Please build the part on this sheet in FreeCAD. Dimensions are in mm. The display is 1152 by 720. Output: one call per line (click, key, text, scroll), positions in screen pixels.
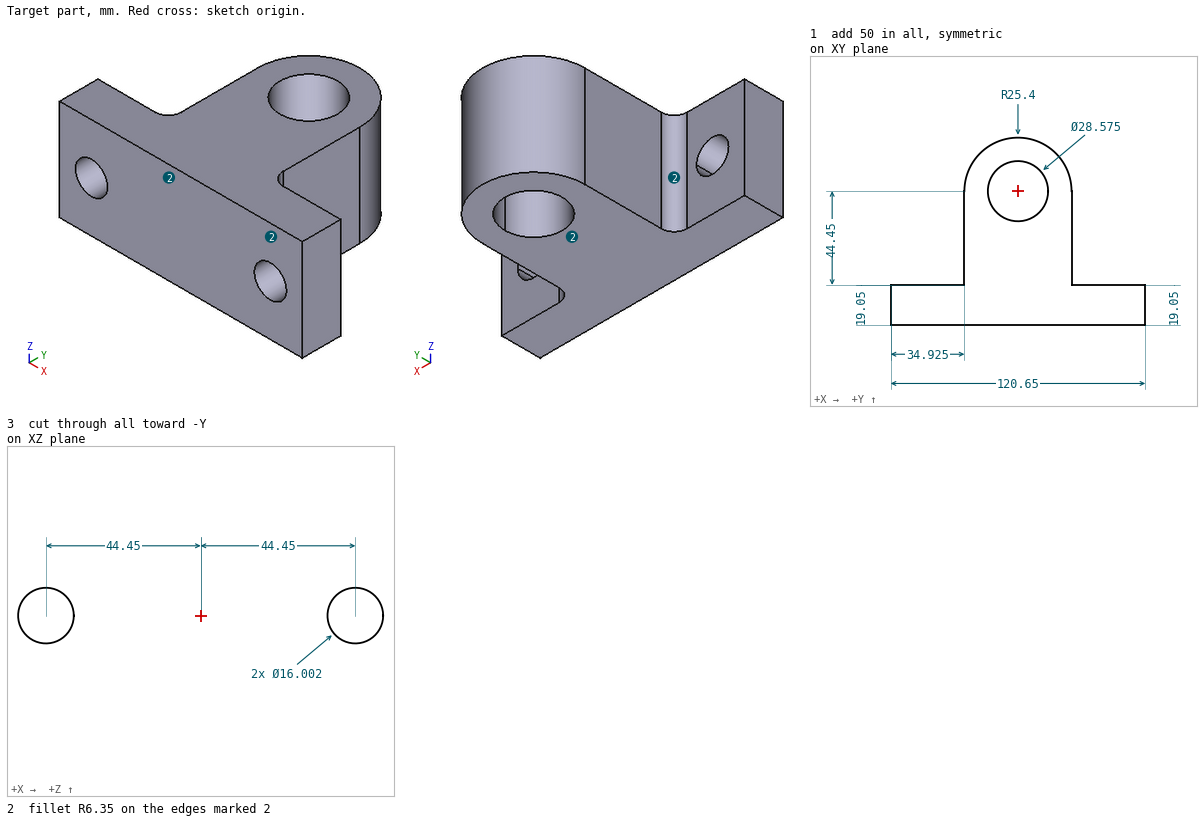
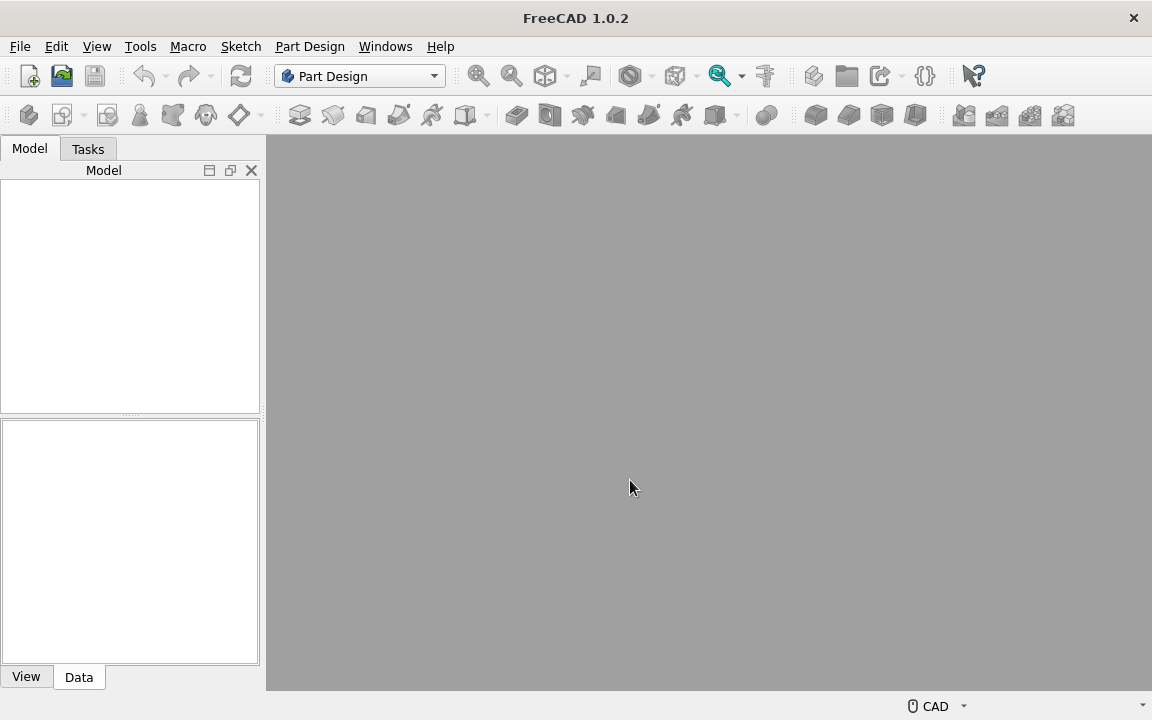
key(ctrl+n)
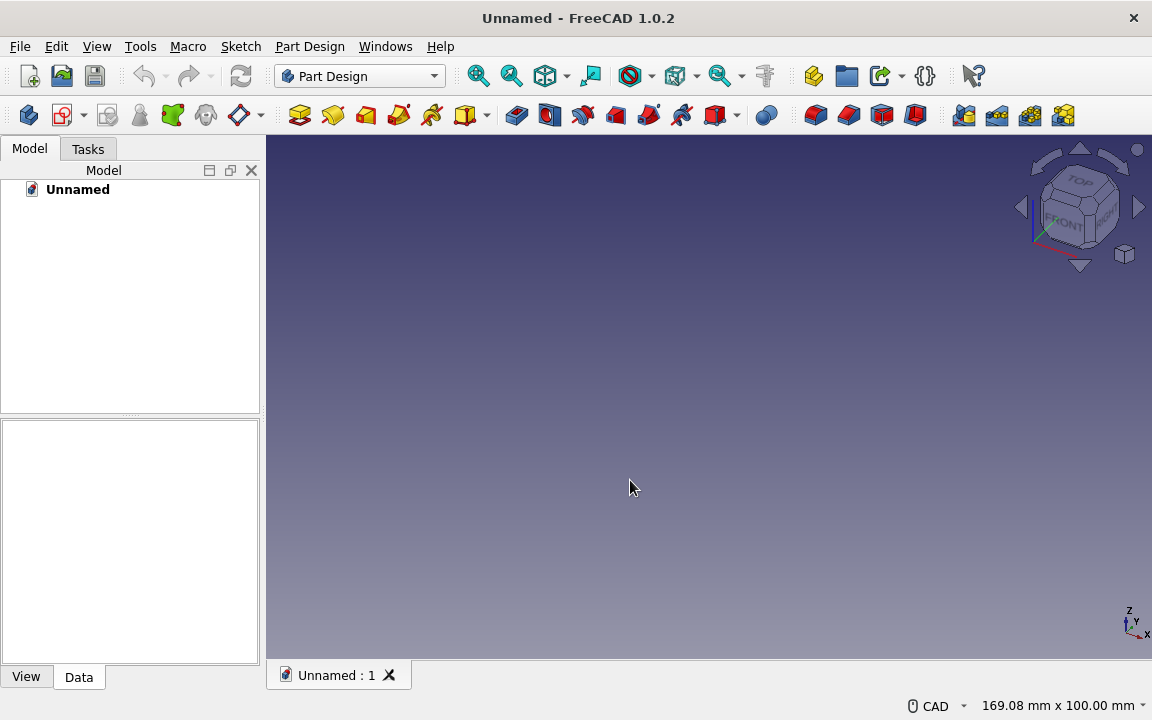
click(62, 116)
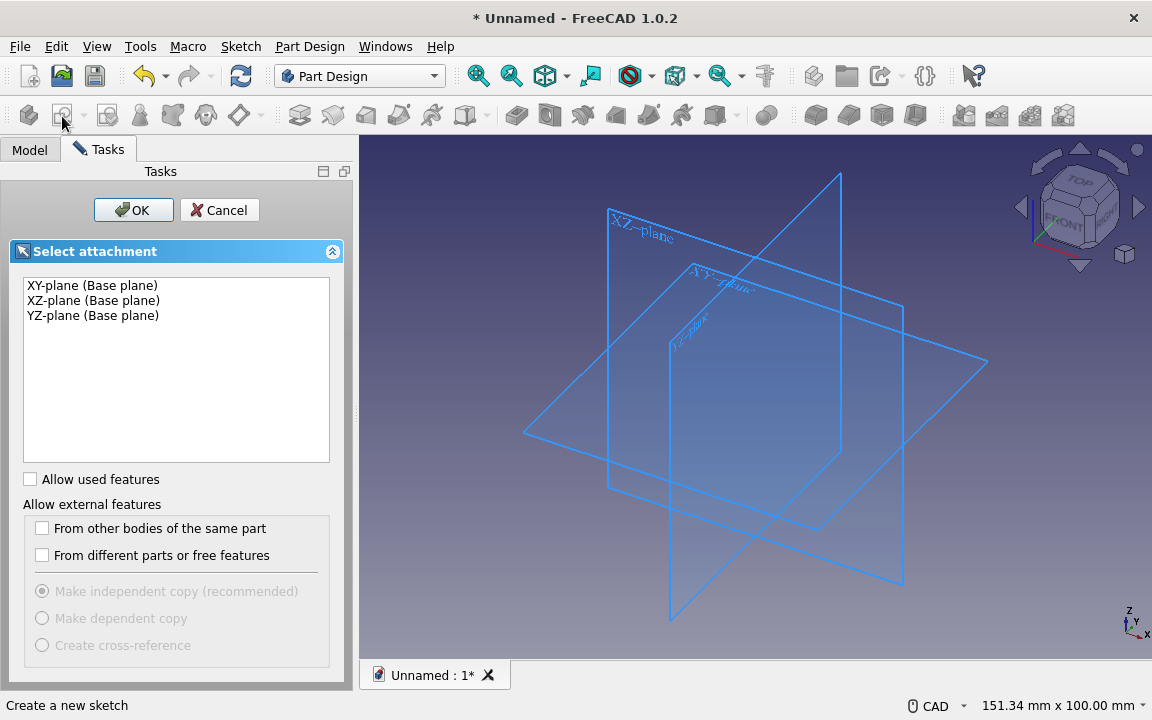
click(84, 286)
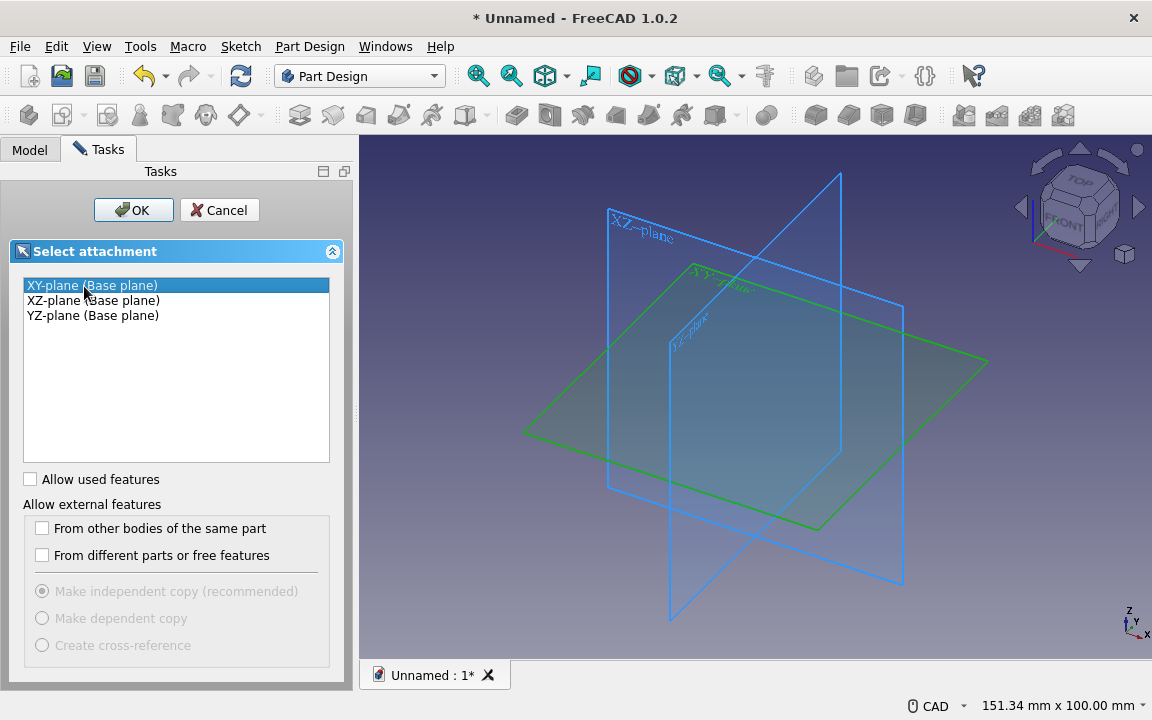
click(134, 210)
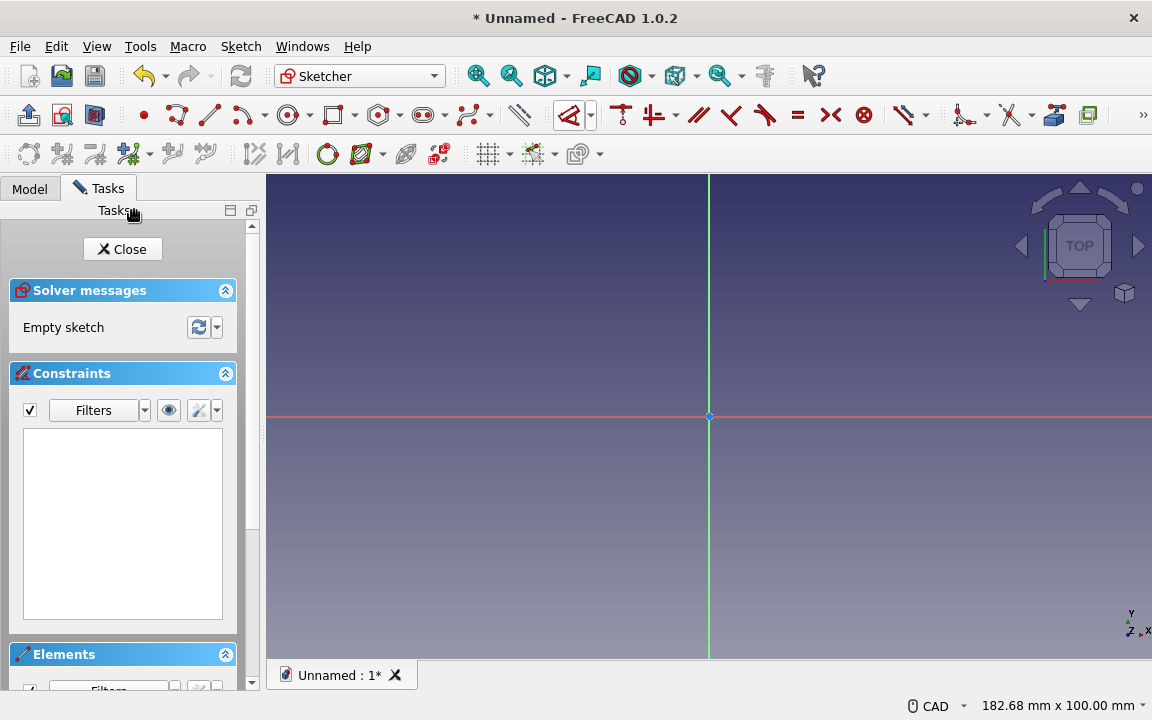
scroll(501, 229, down, 2)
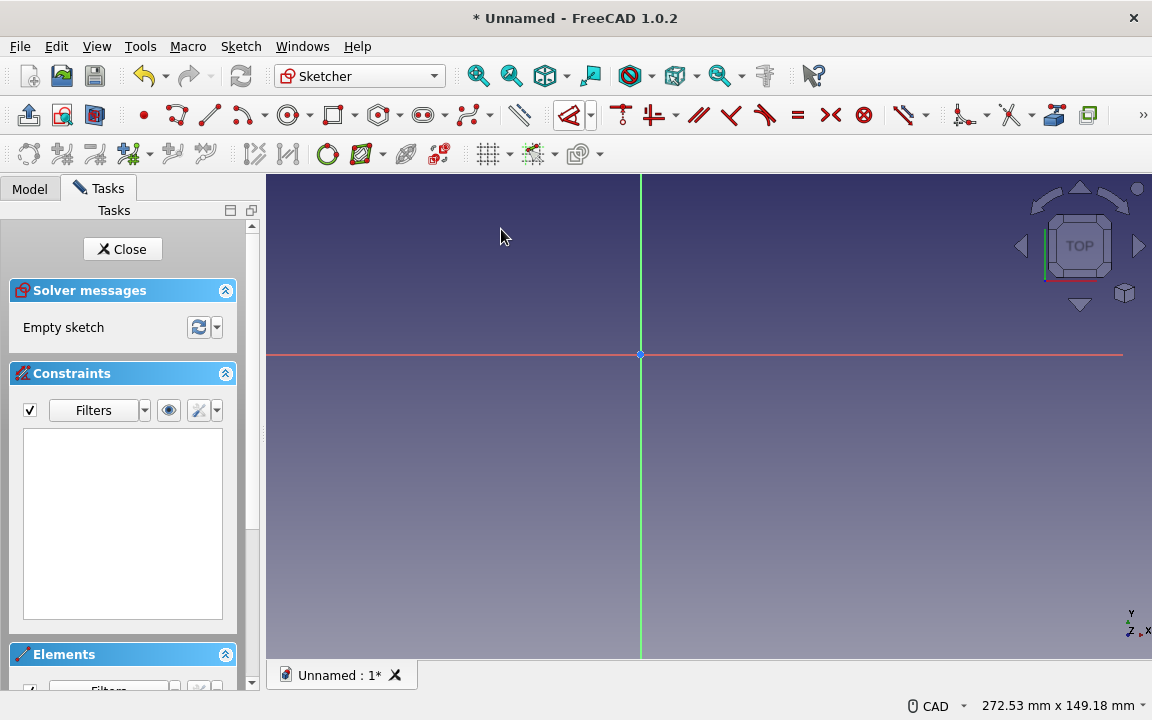
click(177, 116)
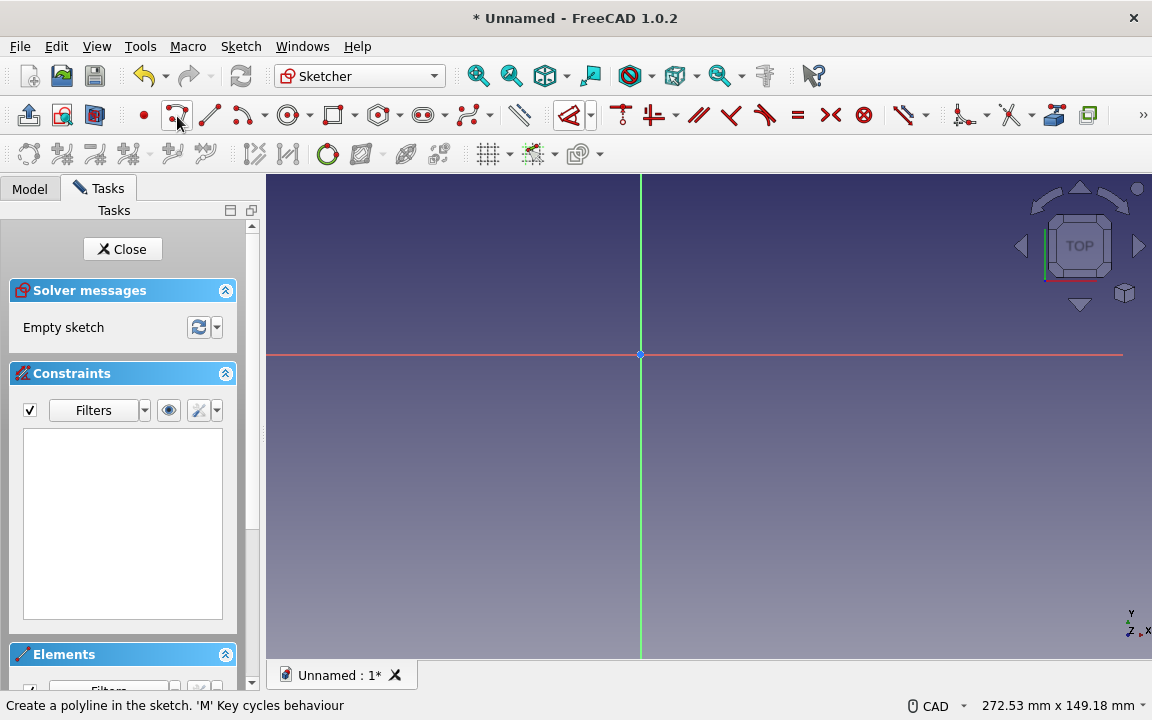
click(558, 355)
click(558, 499)
click(444, 499)
click(444, 561)
click(837, 561)
click(837, 499)
click(723, 499)
click(723, 355)
right_click(723, 355)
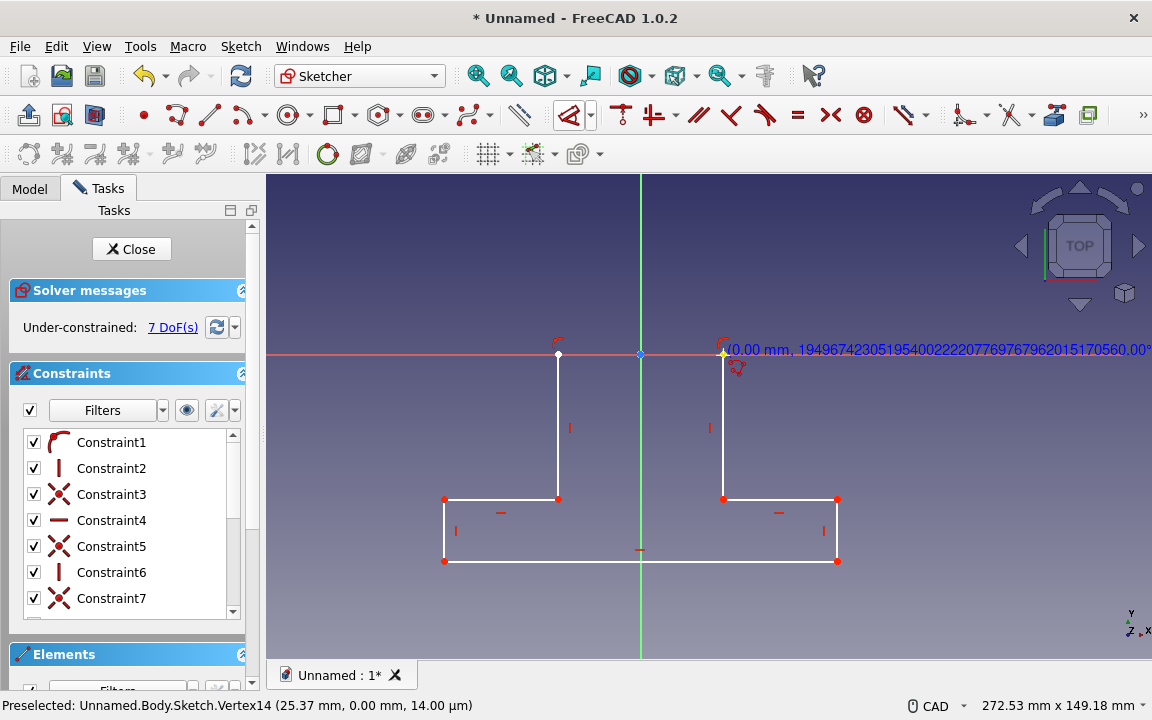
key(g)
key(3)
key(a)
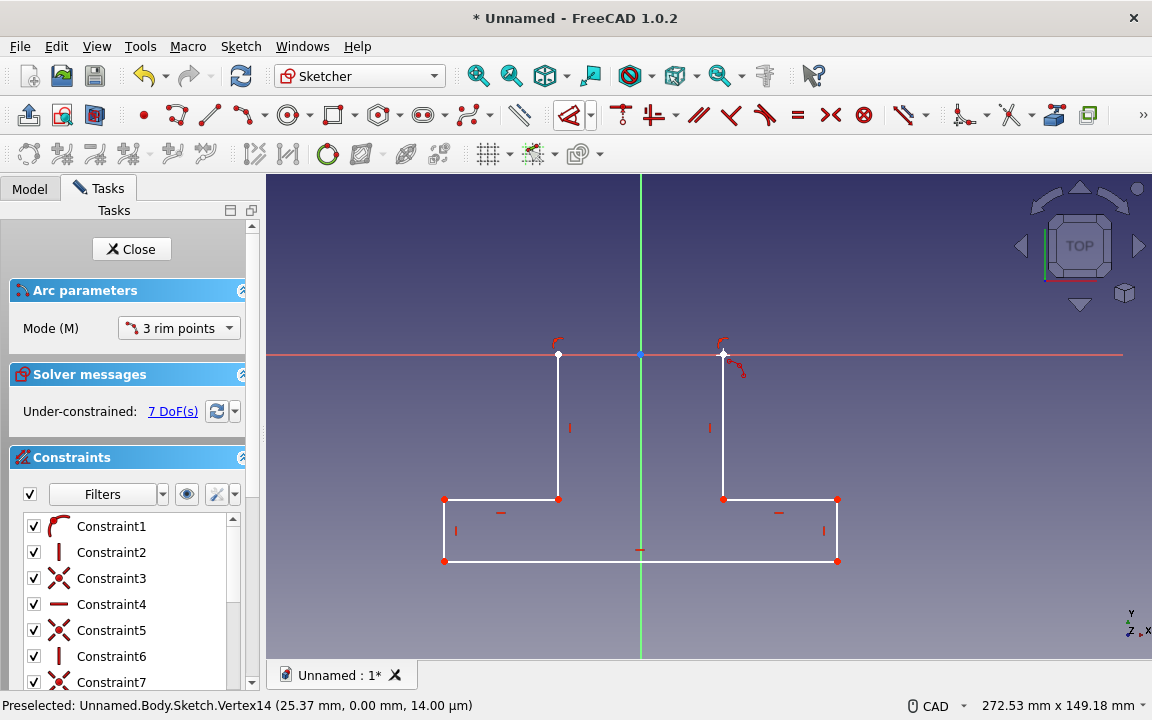
click(723, 355)
click(558, 355)
click(666, 276)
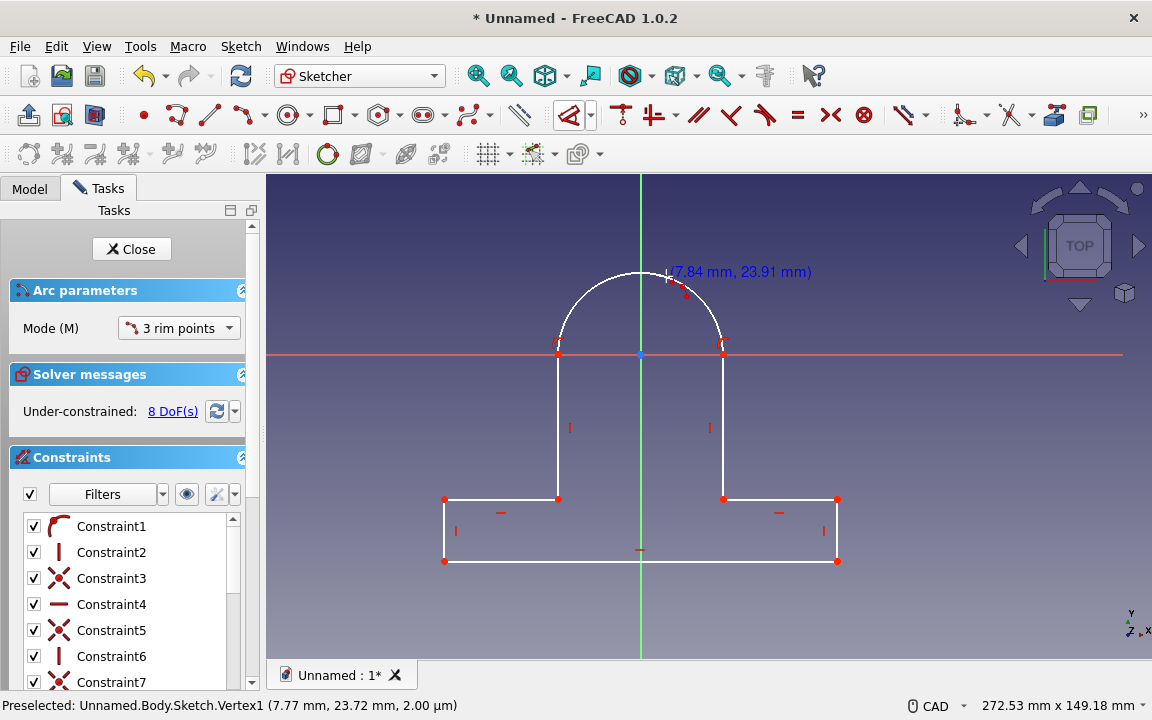
click(288, 116)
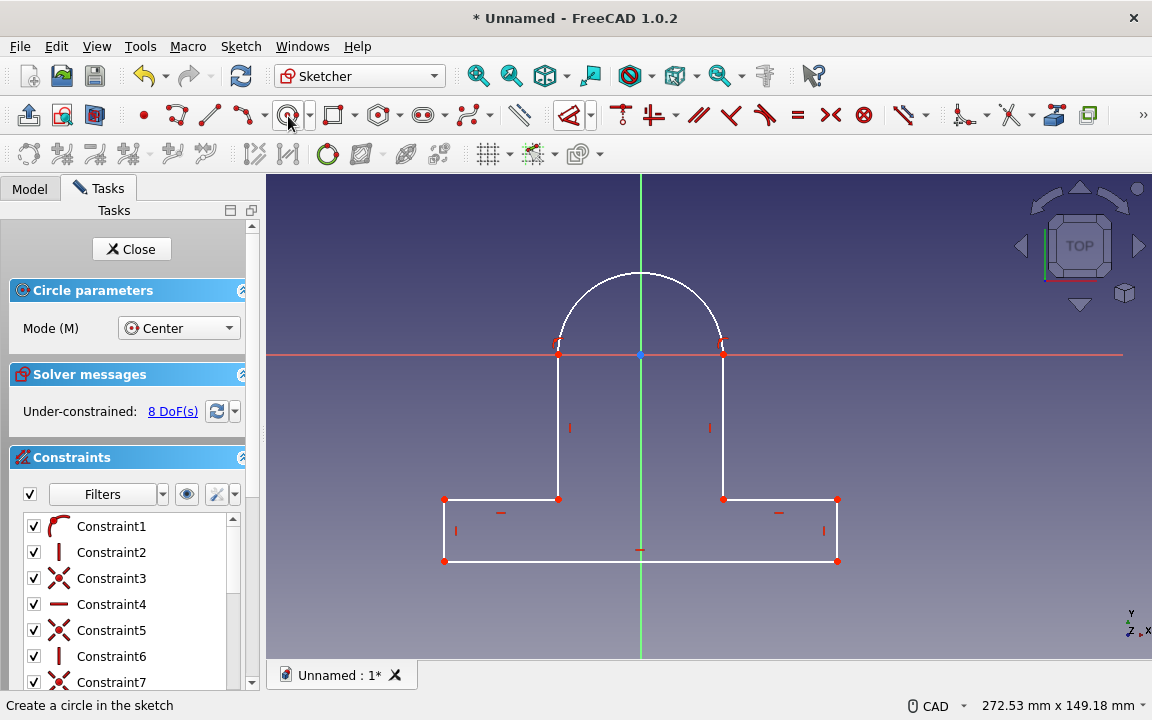
click(641, 355)
move(673, 322)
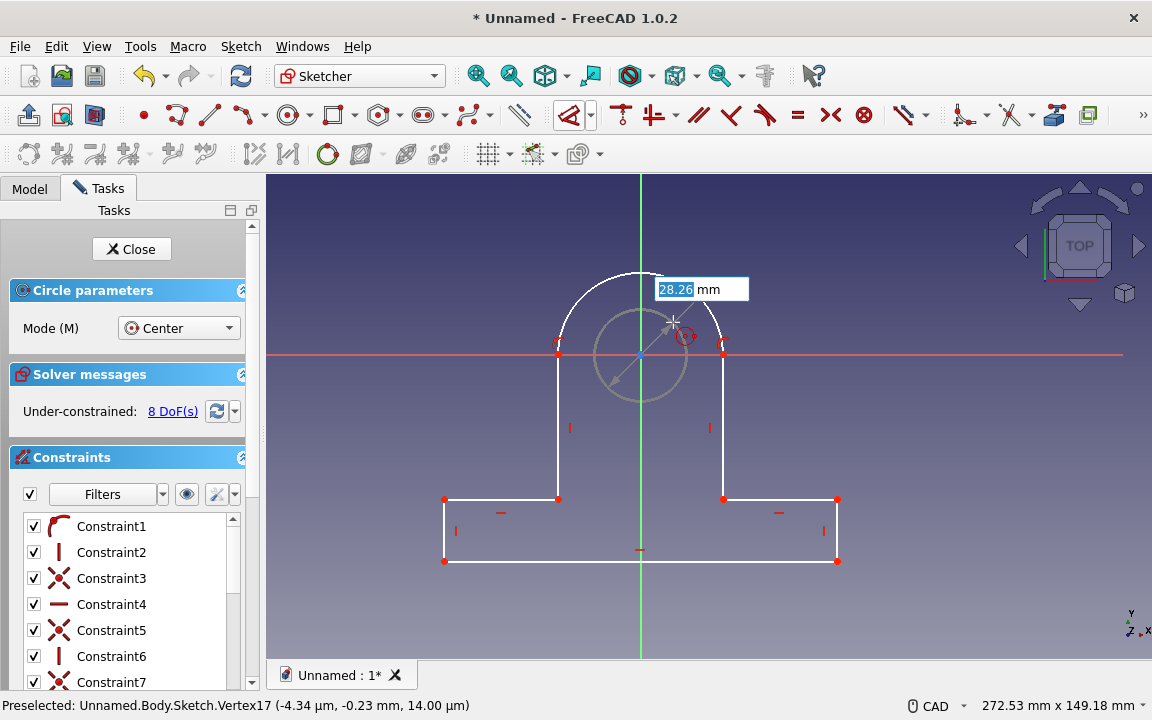
text(28.575)
key(Return)
key(Escape)